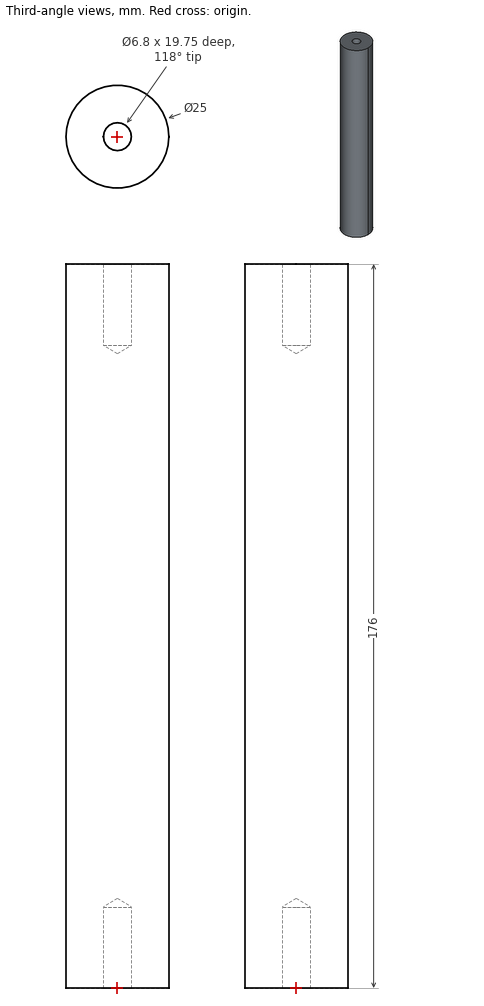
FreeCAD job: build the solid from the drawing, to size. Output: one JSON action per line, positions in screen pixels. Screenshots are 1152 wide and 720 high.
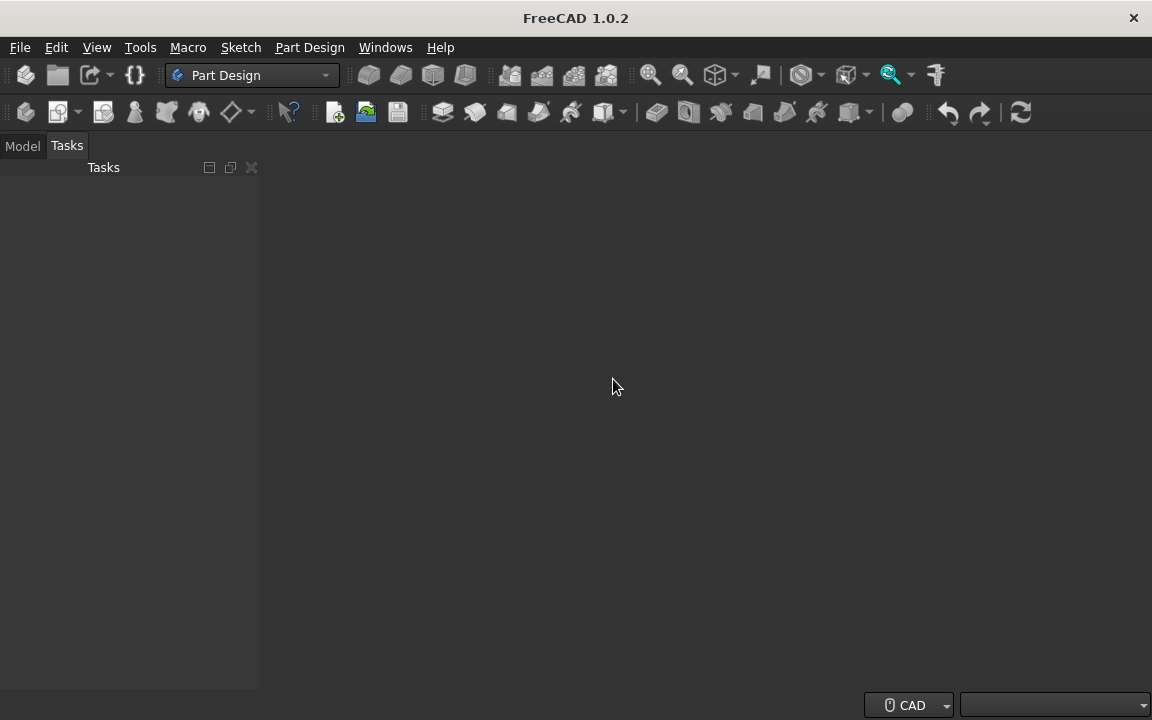
{"action": "left_click", "coordinate": [334, 112]}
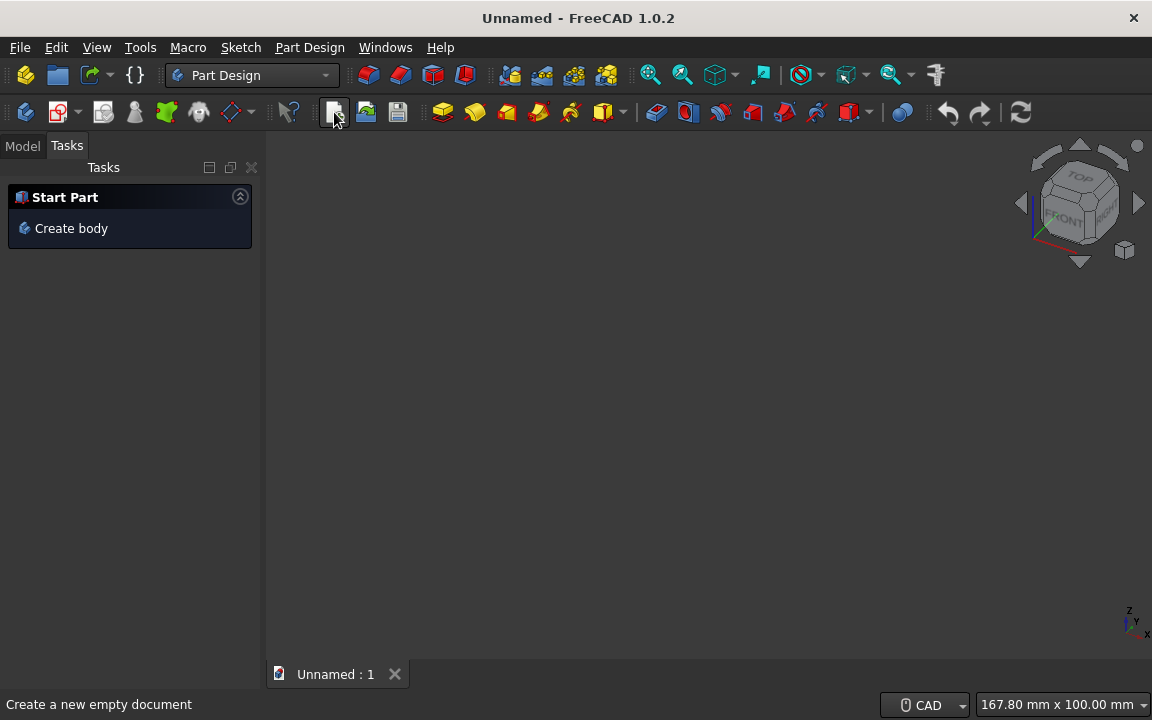
{"action": "left_click", "coordinate": [58, 112]}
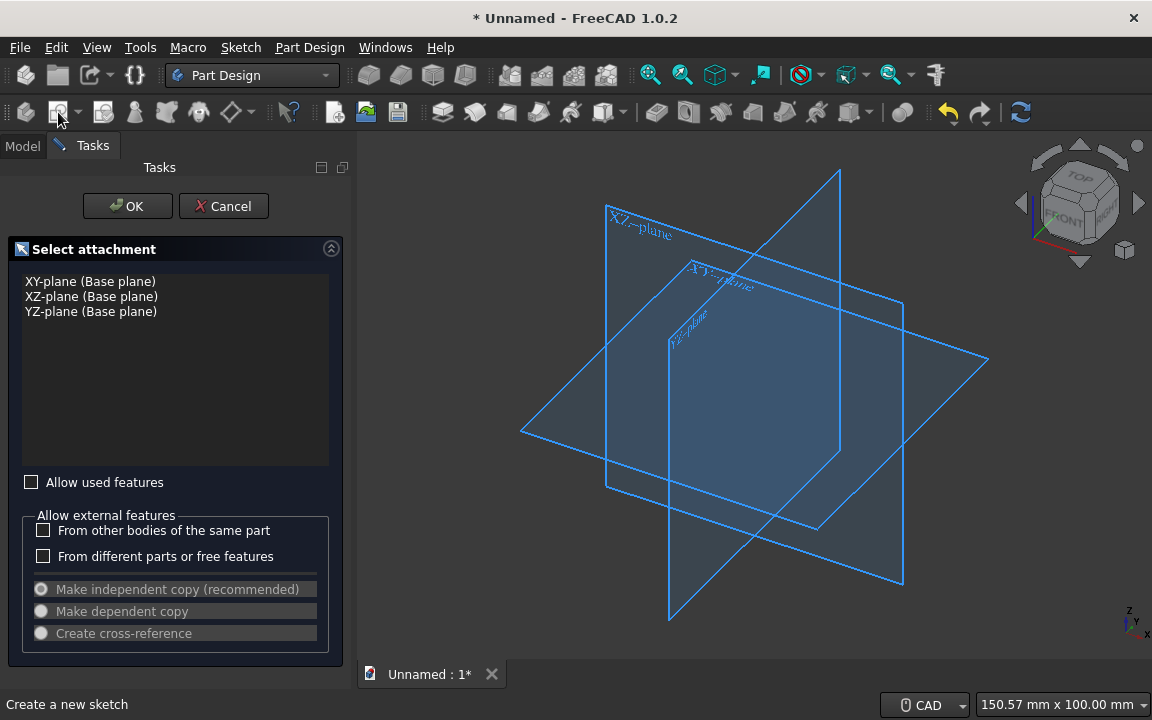
{"action": "left_click", "coordinate": [82, 282]}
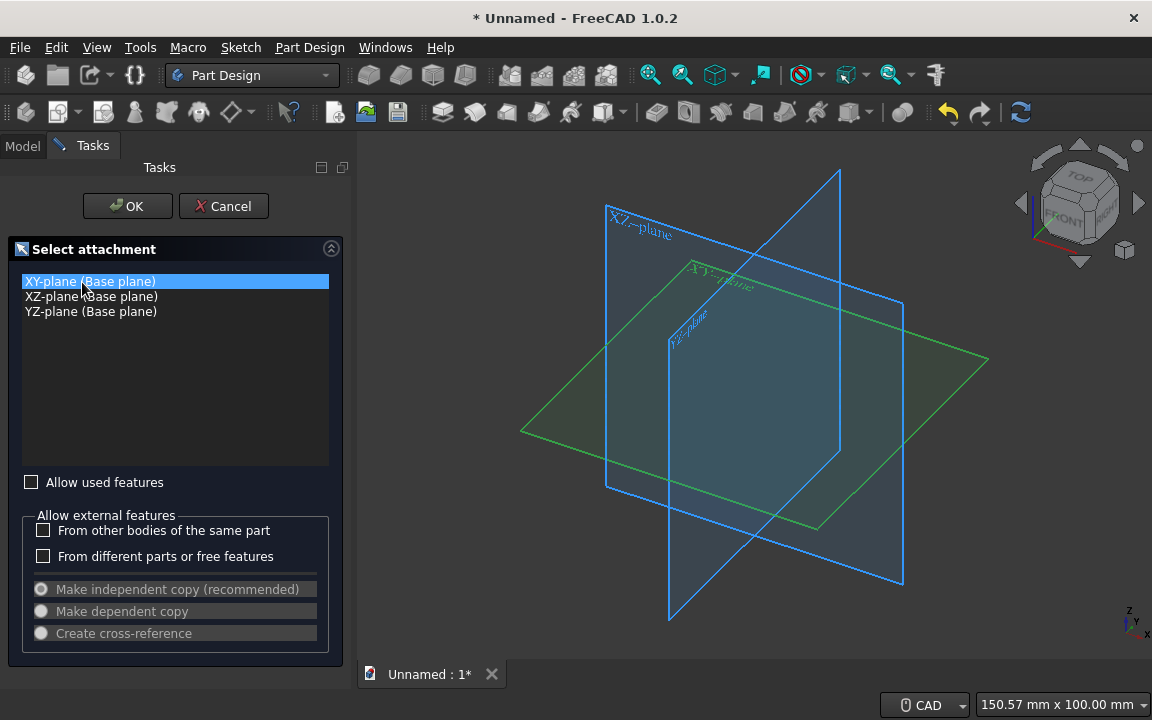
{"action": "left_click", "coordinate": [128, 206]}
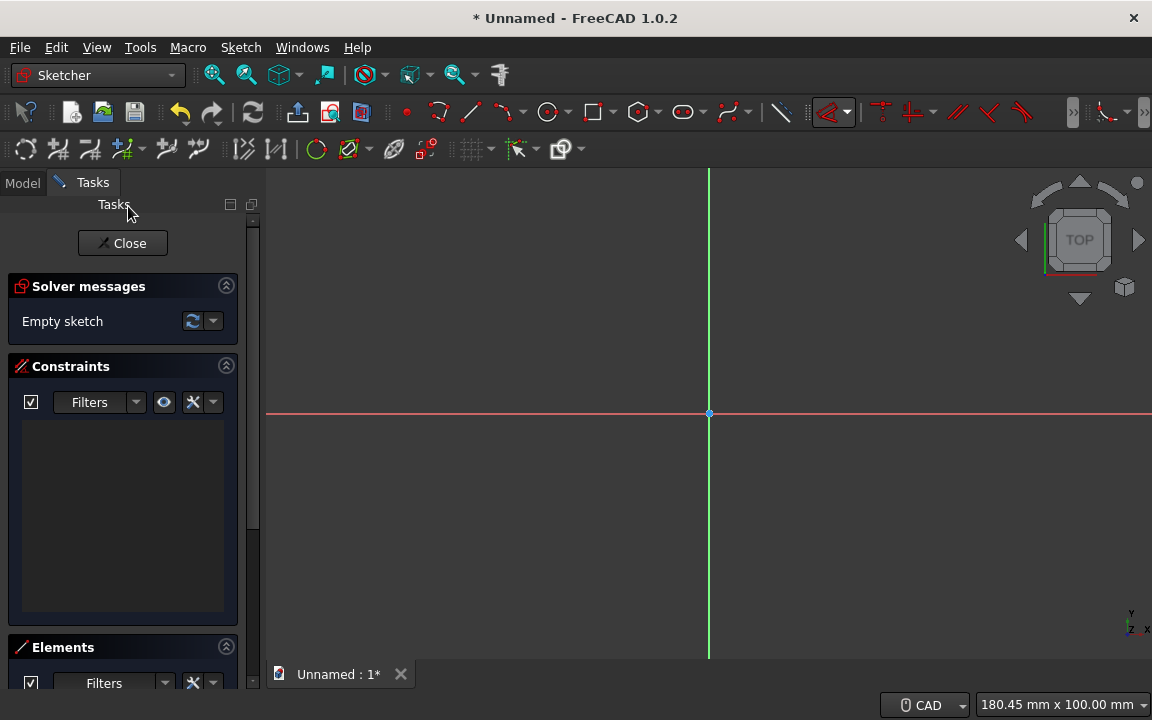
{"action": "scroll", "coordinate": [749, 414], "scroll_direction": "up", "scroll_amount": 5}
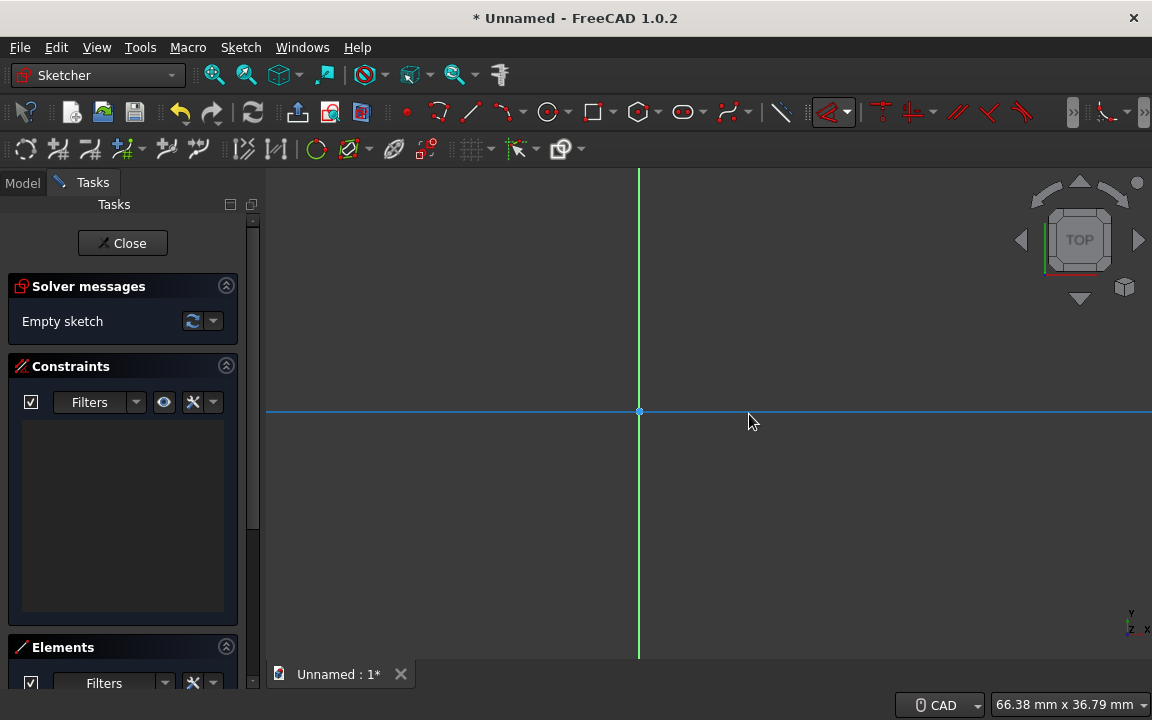
{"action": "left_click", "coordinate": [548, 112]}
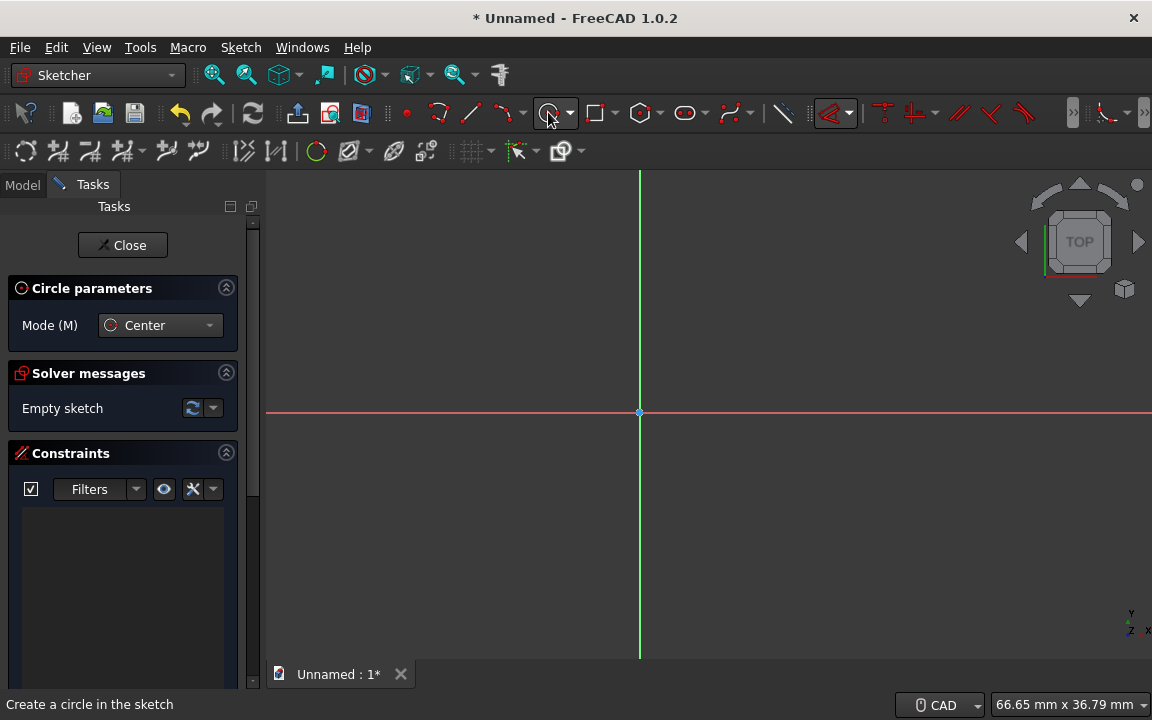
{"action": "left_click", "coordinate": [640, 413]}
{"action": "left_click", "coordinate": [757, 295]}
{"action": "key", "text": "Escape"}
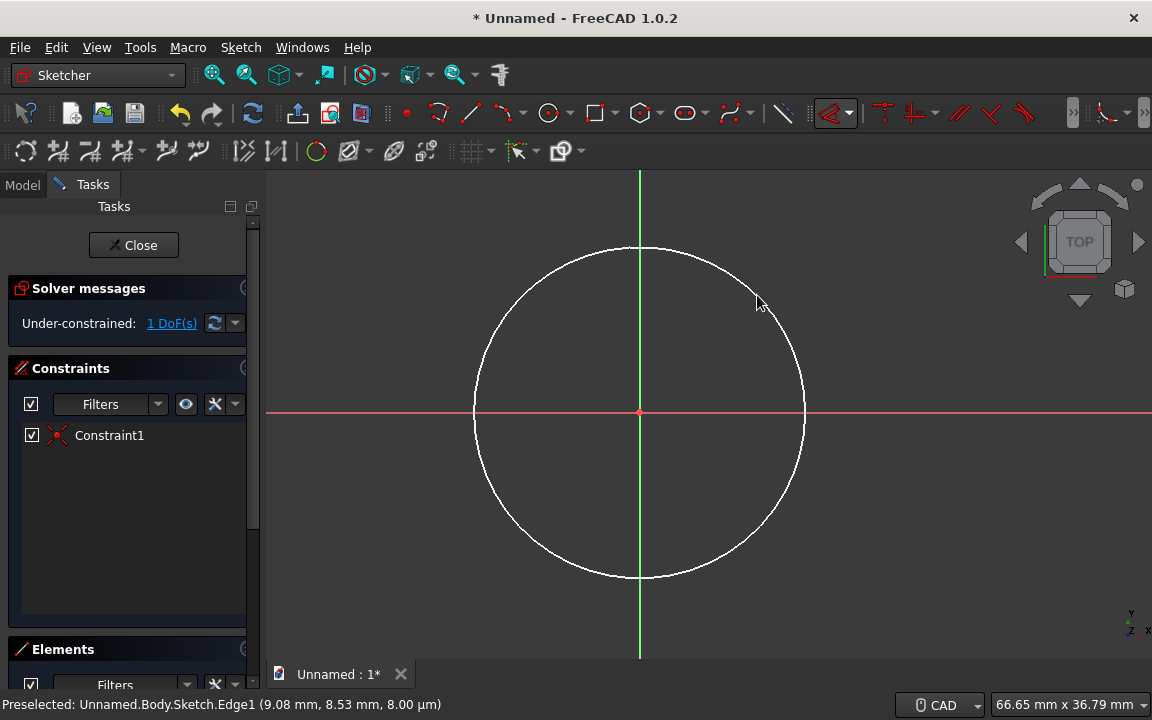
{"action": "left_click", "coordinate": [830, 114]}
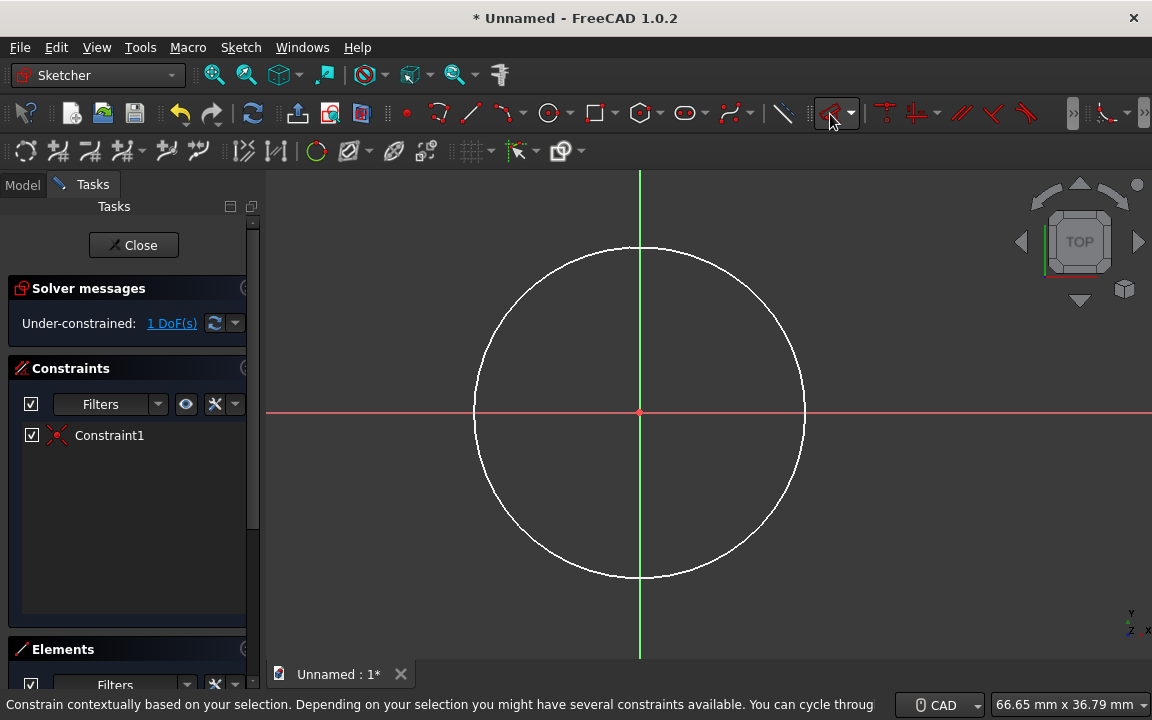
{"action": "left_click", "coordinate": [756, 295]}
{"action": "left_click", "coordinate": [778, 272]}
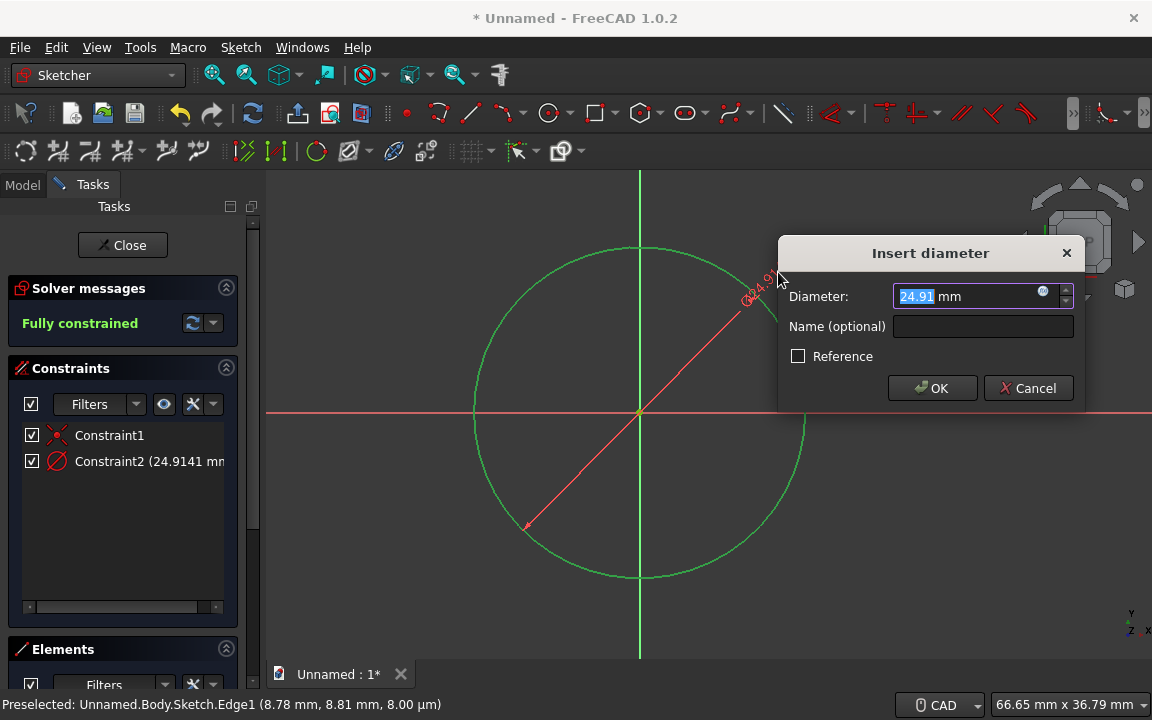
{"action": "type", "text": "25"}
{"action": "key", "text": "Return"}
{"action": "key", "text": "Escape"}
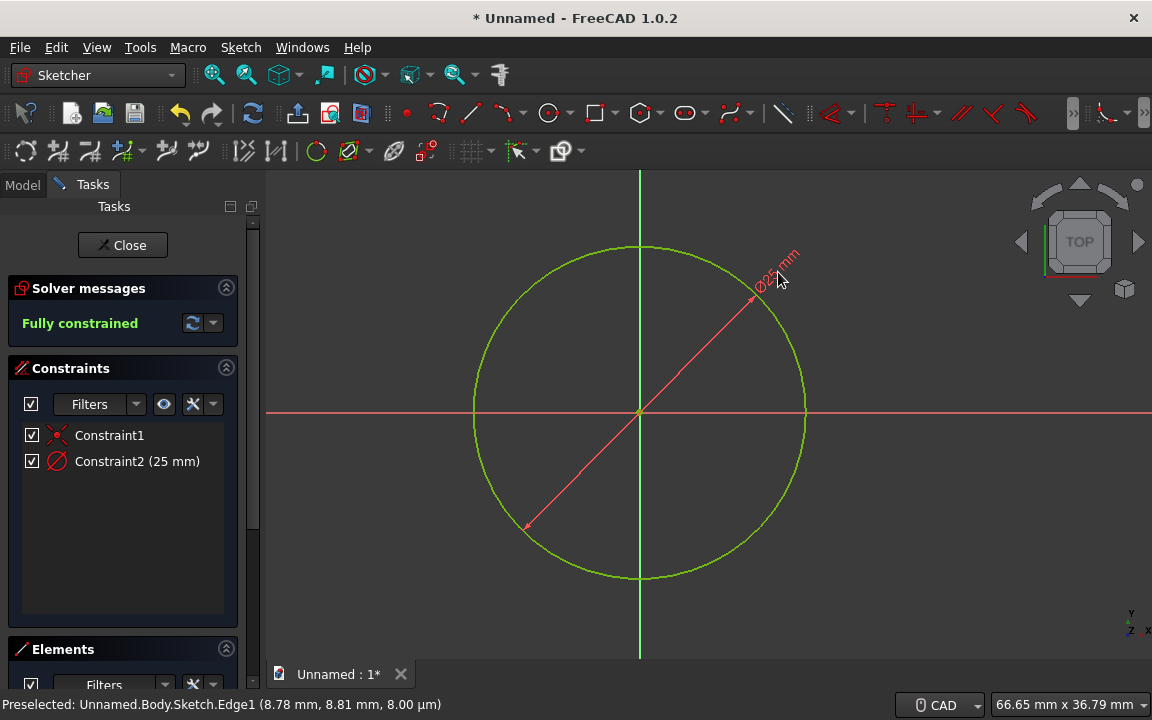
{"action": "left_click", "coordinate": [123, 245]}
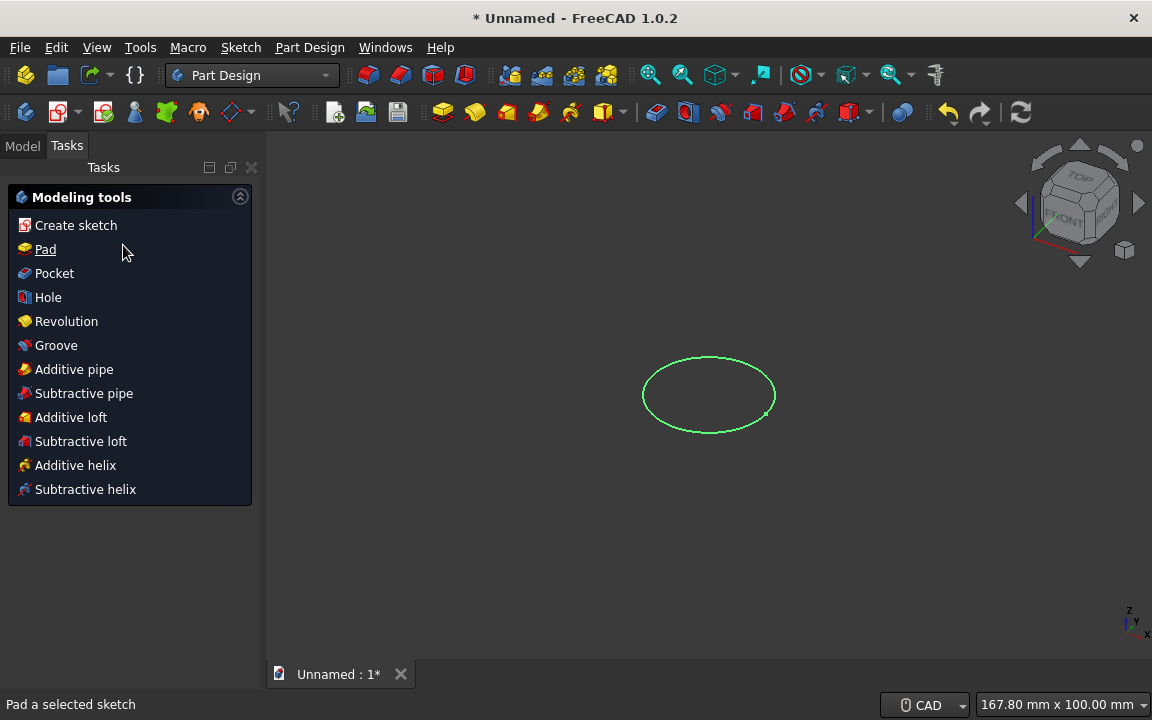
{"action": "left_click", "coordinate": [444, 112]}